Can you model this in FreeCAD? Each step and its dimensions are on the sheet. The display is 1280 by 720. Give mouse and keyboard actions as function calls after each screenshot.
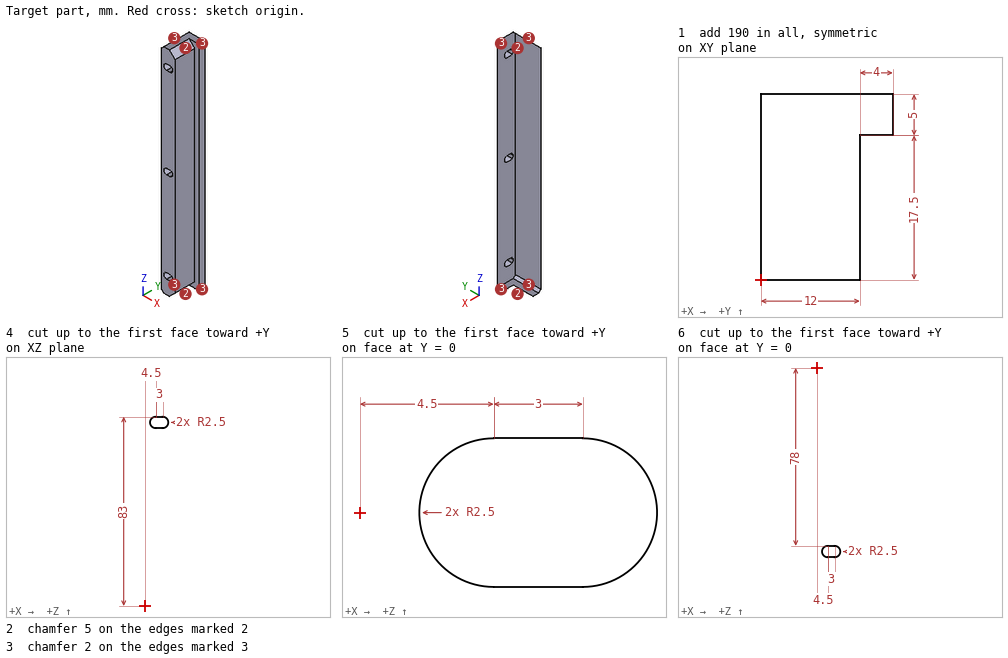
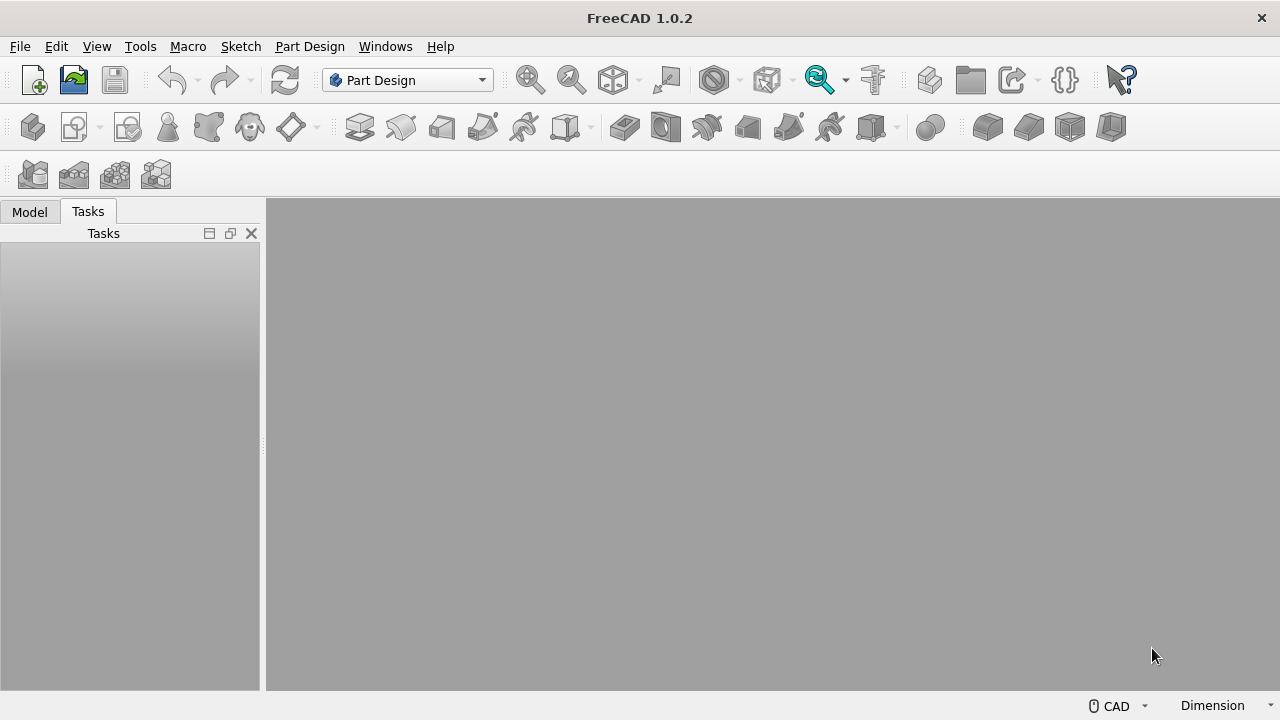
click(33, 80)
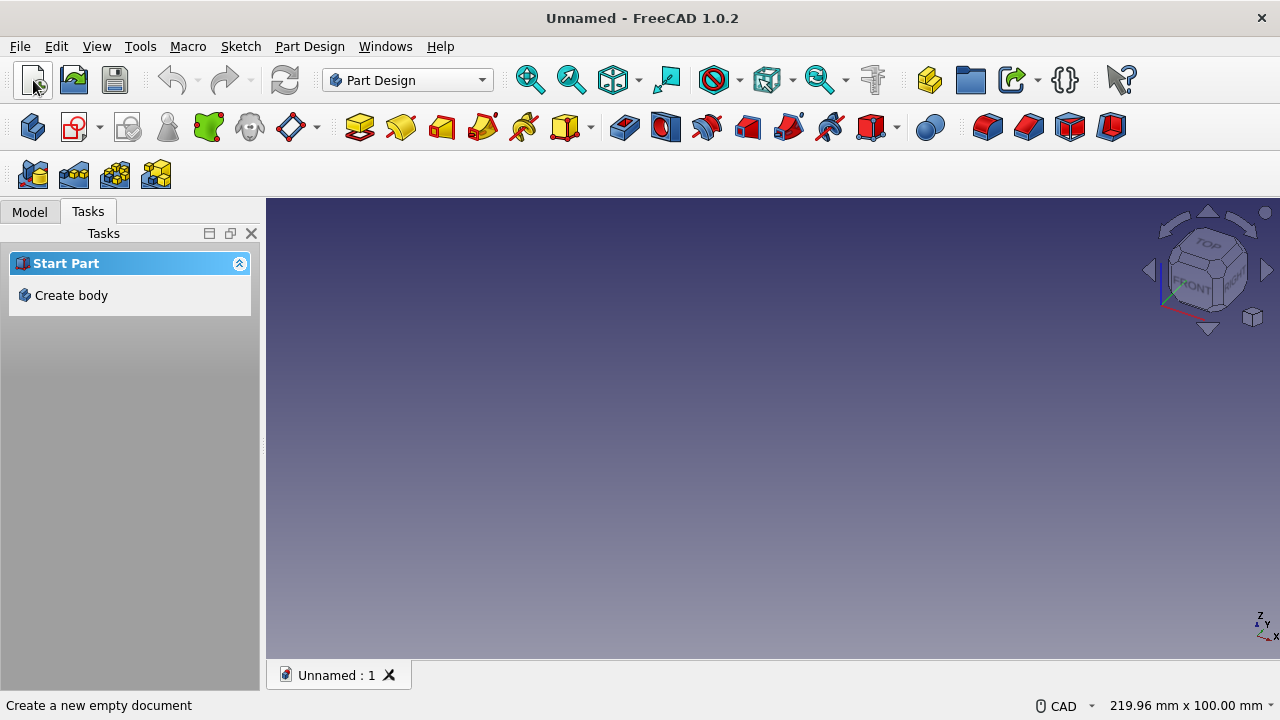
click(74, 128)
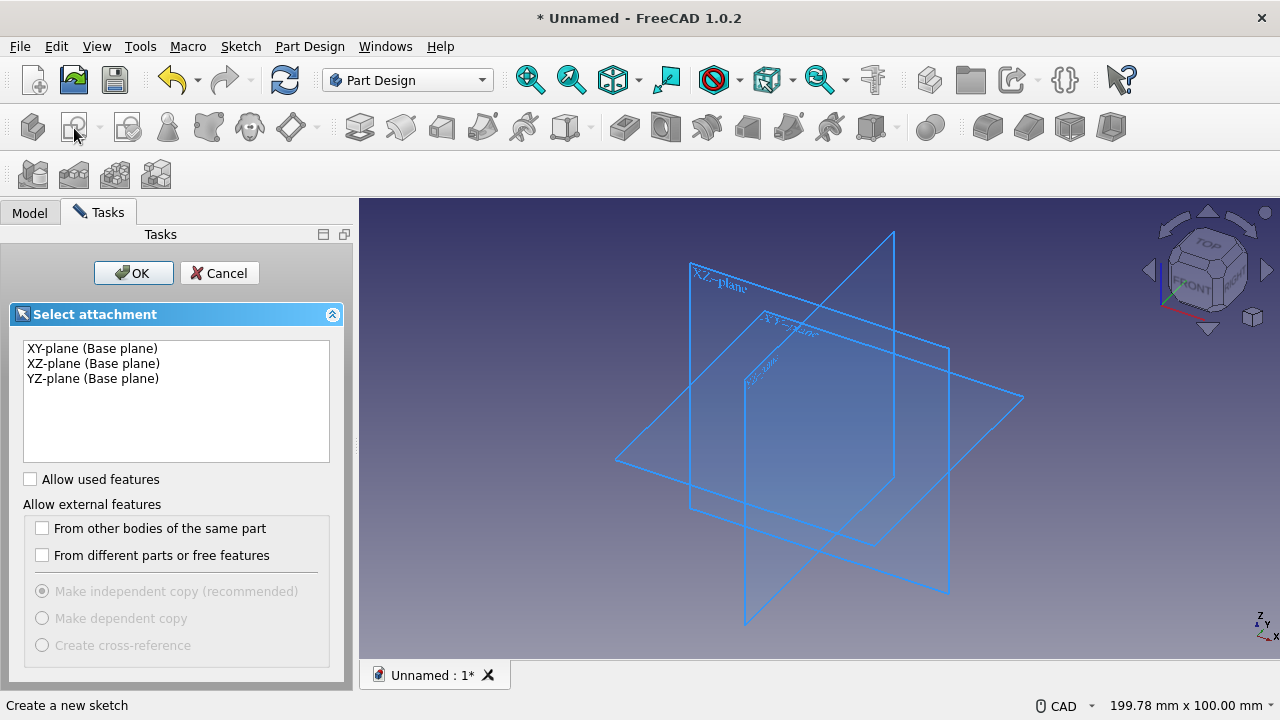
click(84, 348)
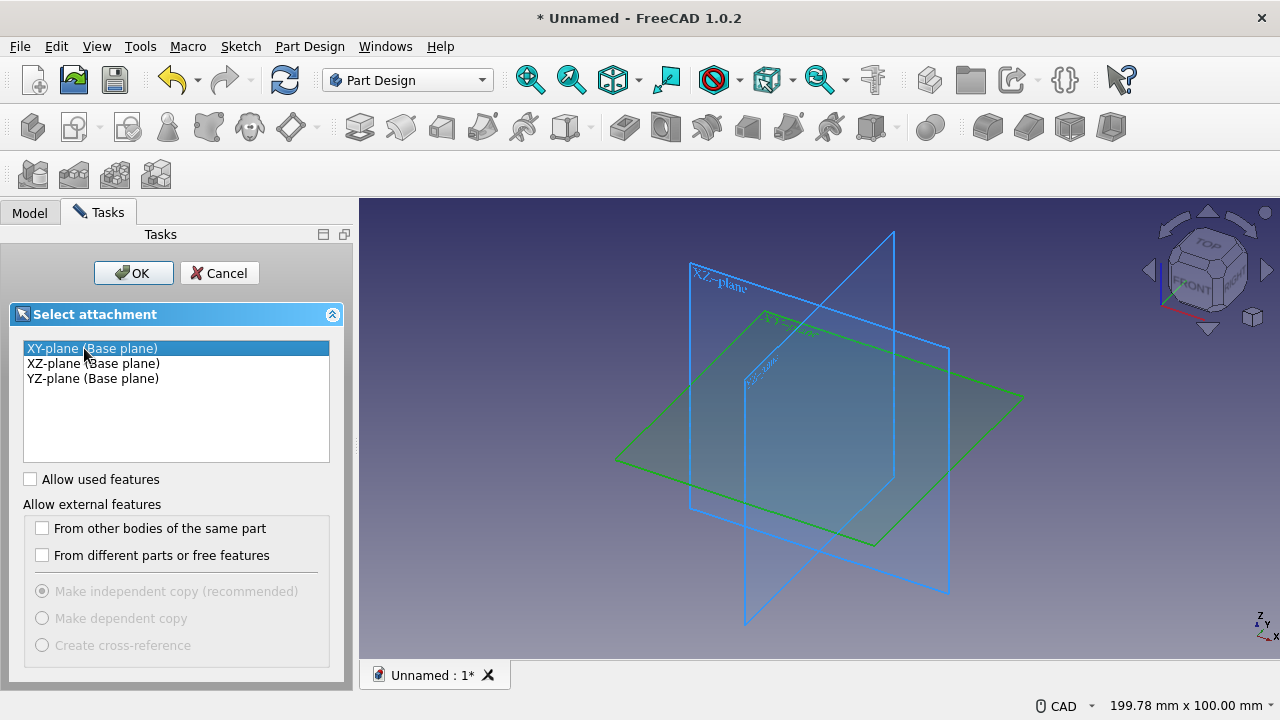
click(134, 273)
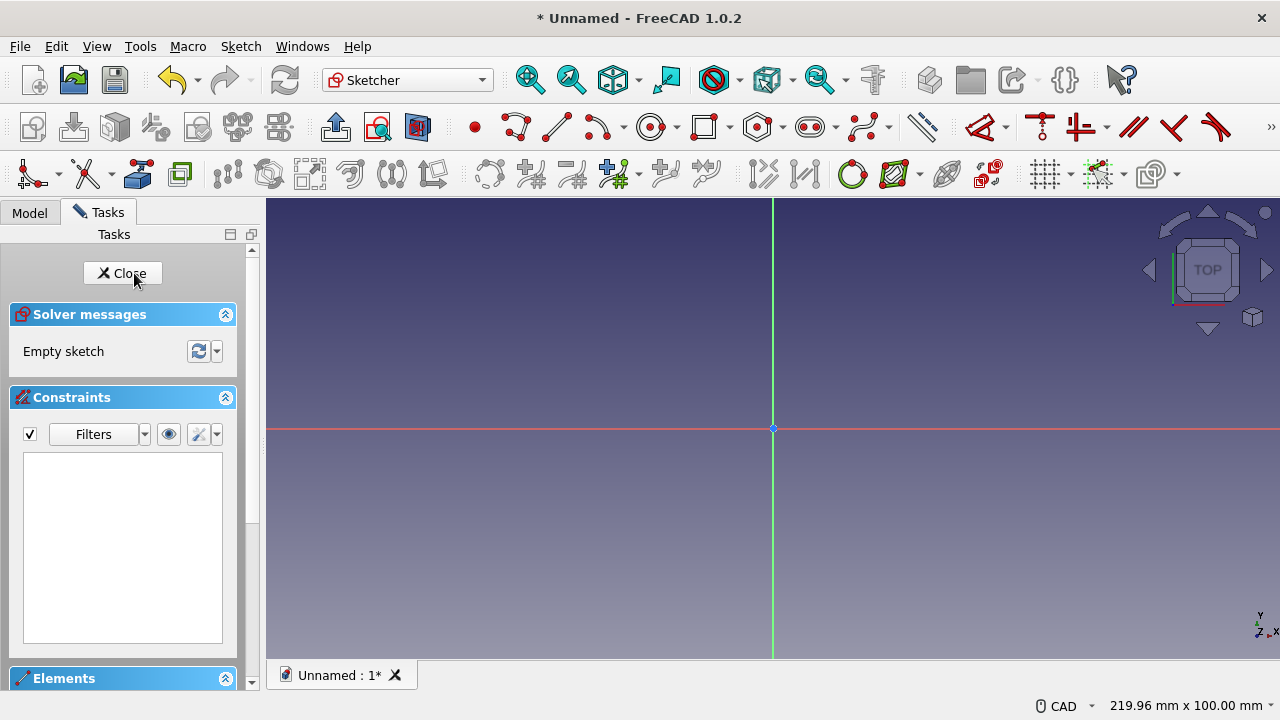
scroll(871, 346, up, 5)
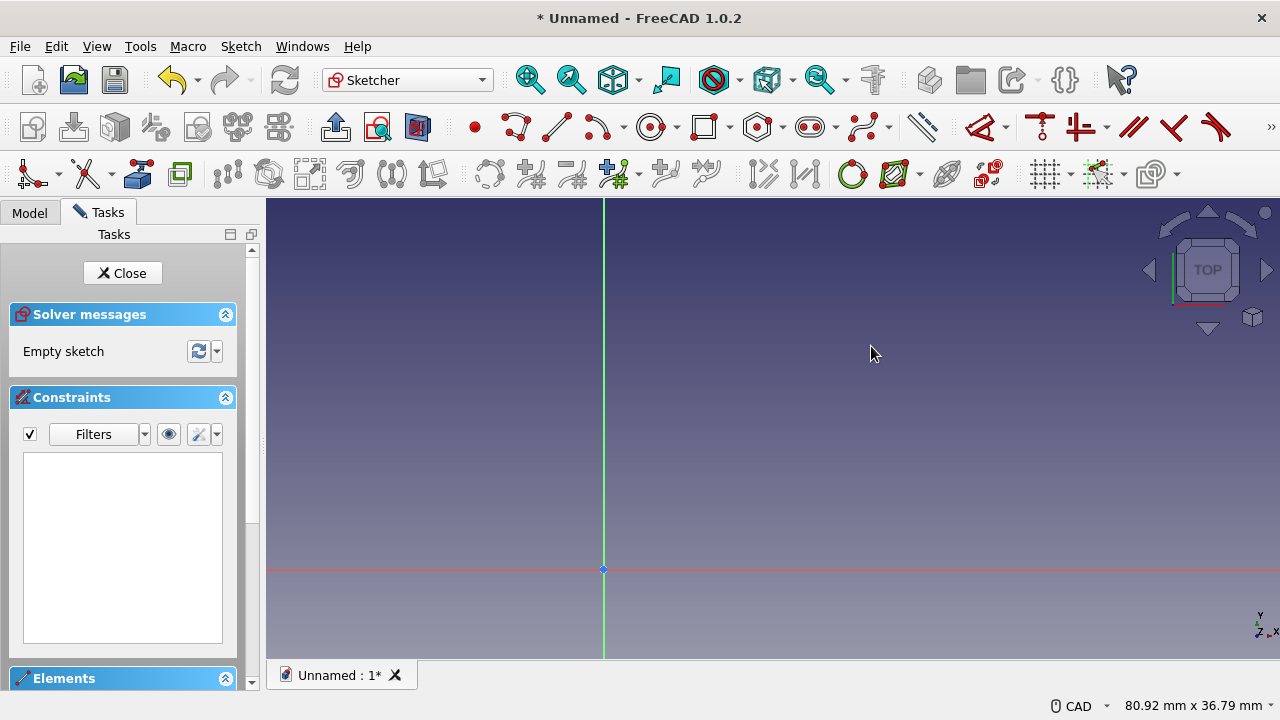
click(516, 128)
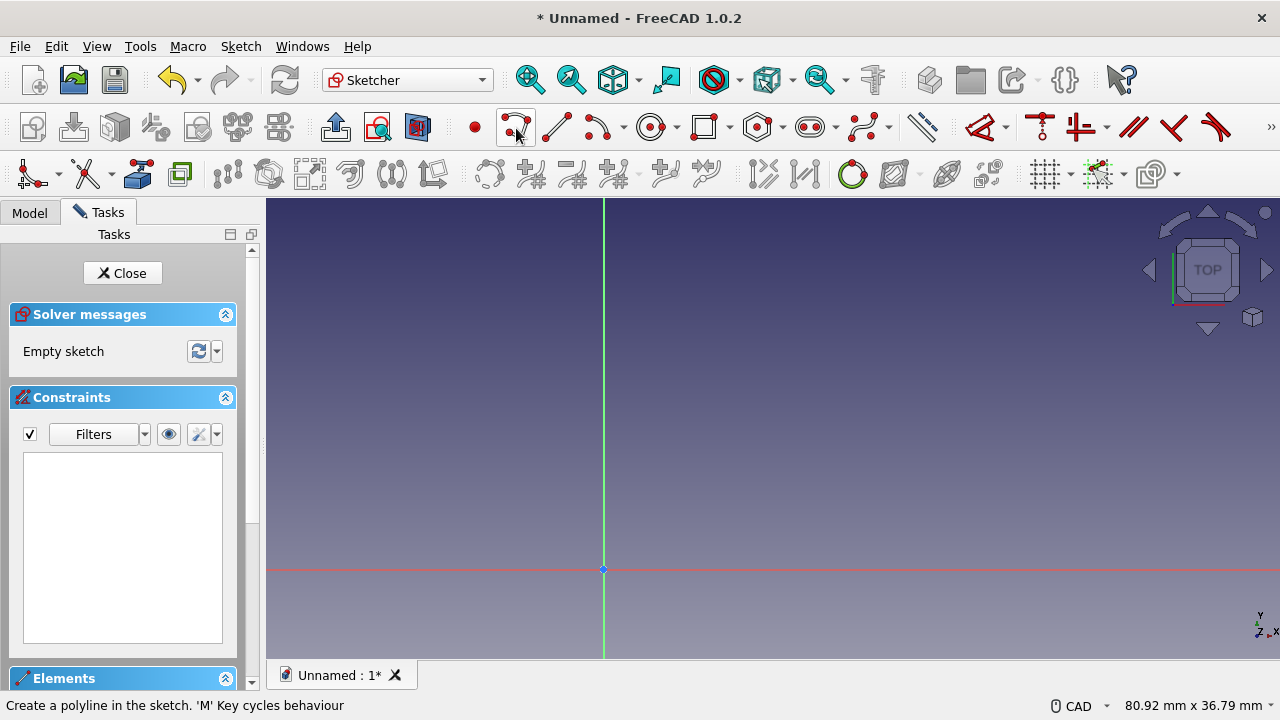
click(604, 570)
click(754, 561)
click(754, 350)
click(804, 350)
click(804, 288)
click(613, 288)
click(604, 570)
key(Escape)
key(Escape)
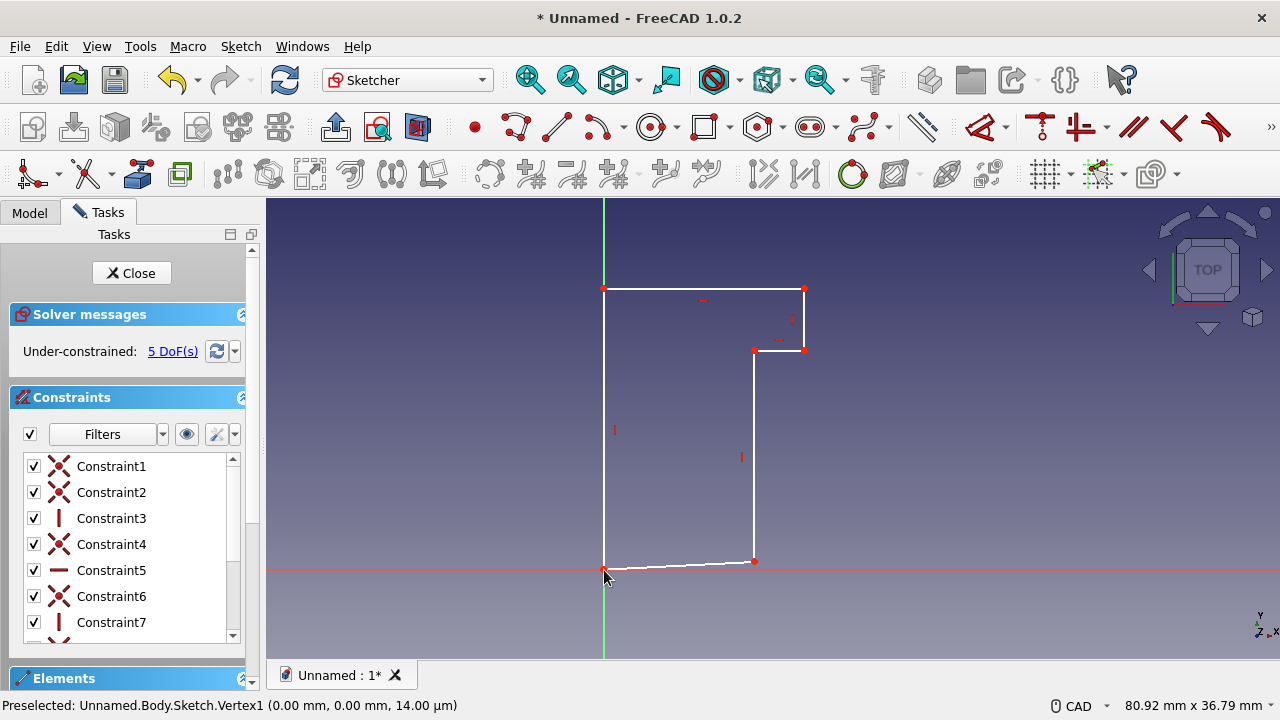
click(649, 567)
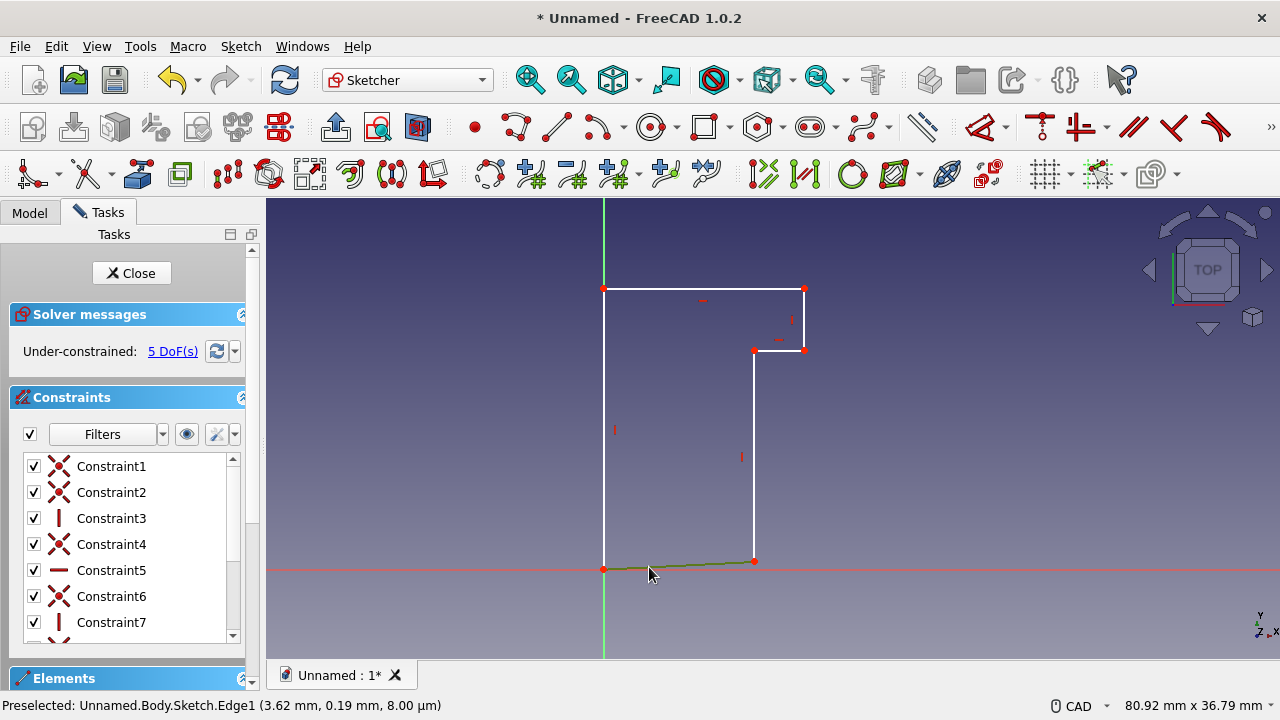
click(1106, 128)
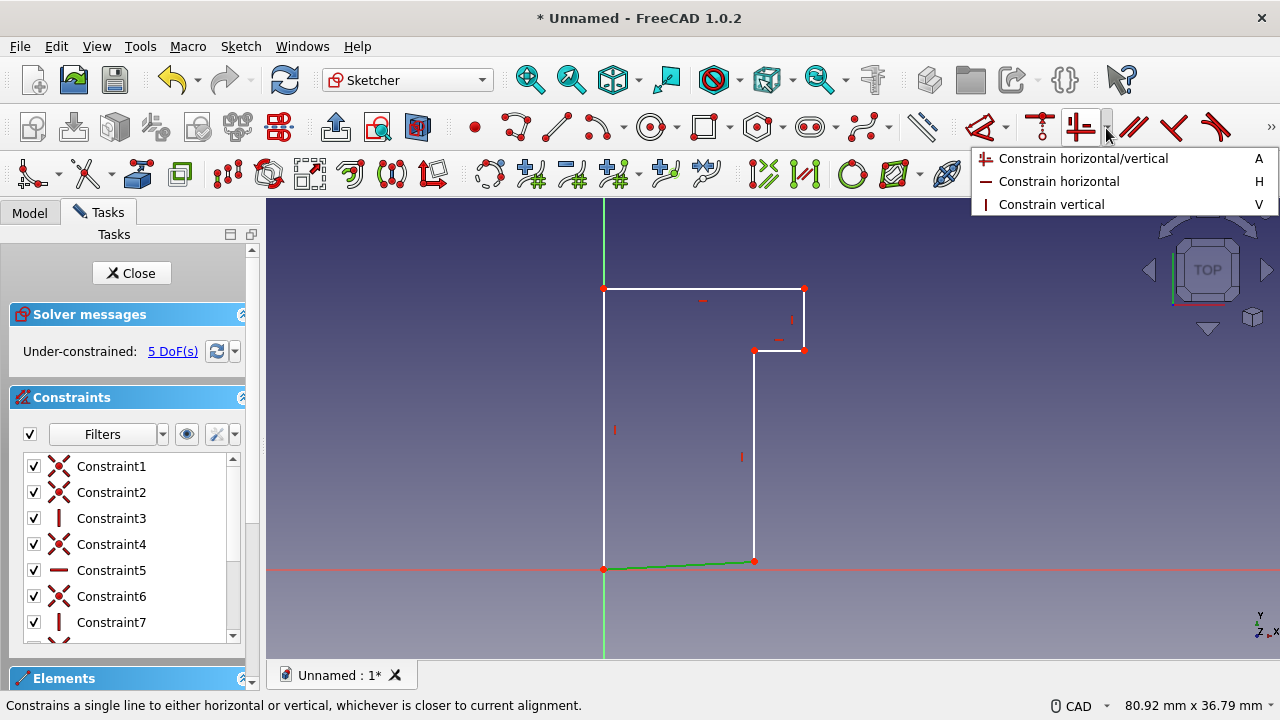
click(1125, 182)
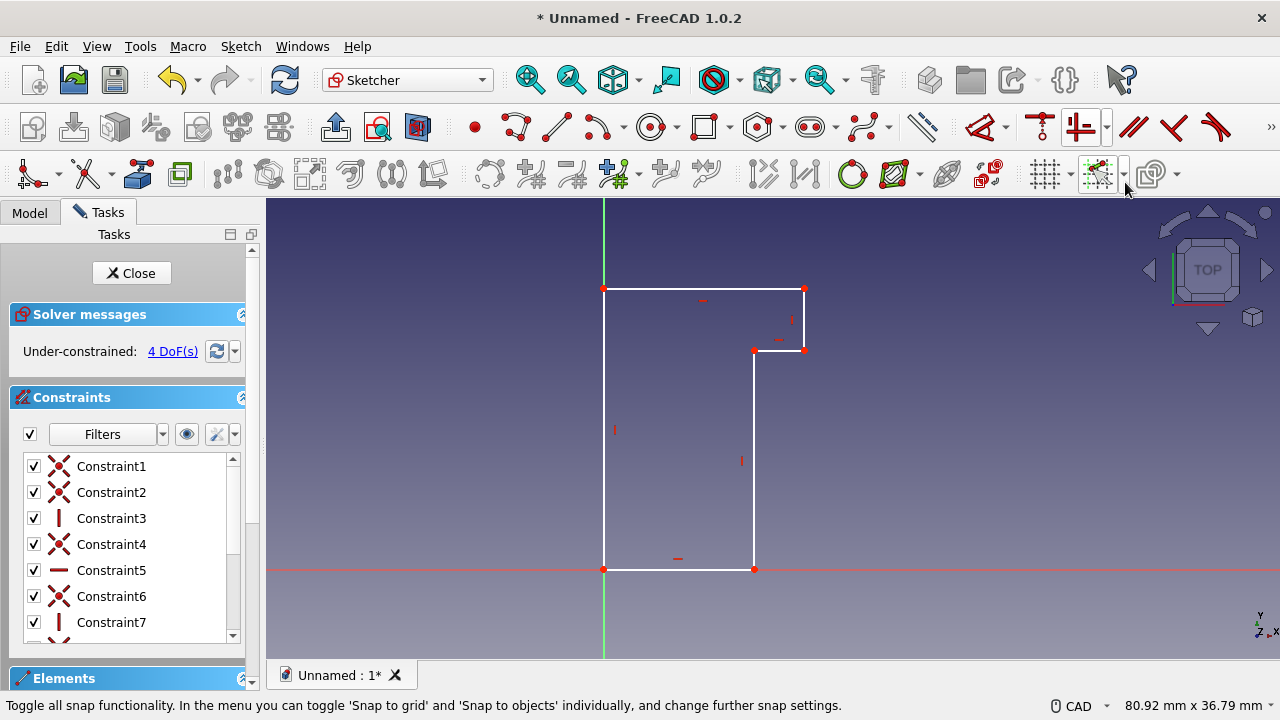
click(980, 128)